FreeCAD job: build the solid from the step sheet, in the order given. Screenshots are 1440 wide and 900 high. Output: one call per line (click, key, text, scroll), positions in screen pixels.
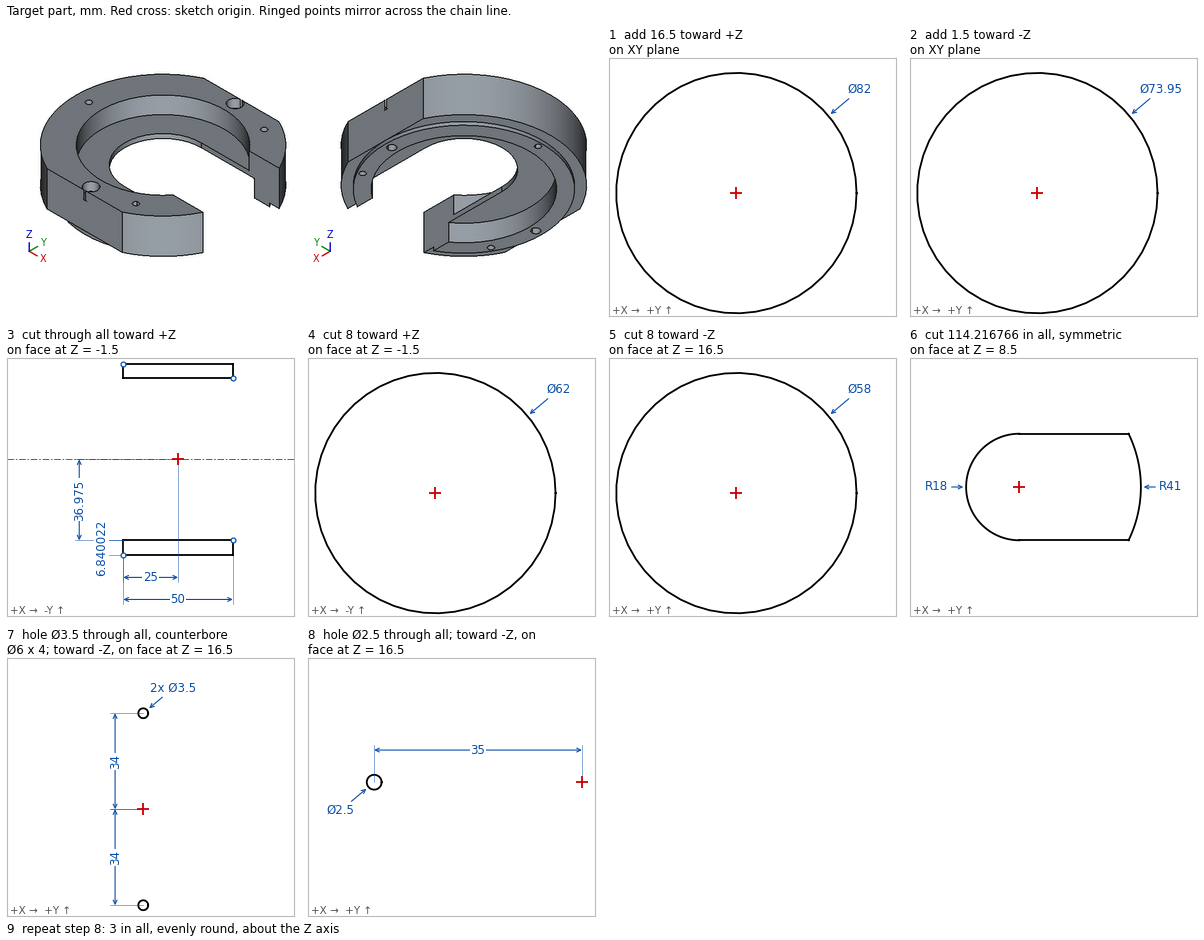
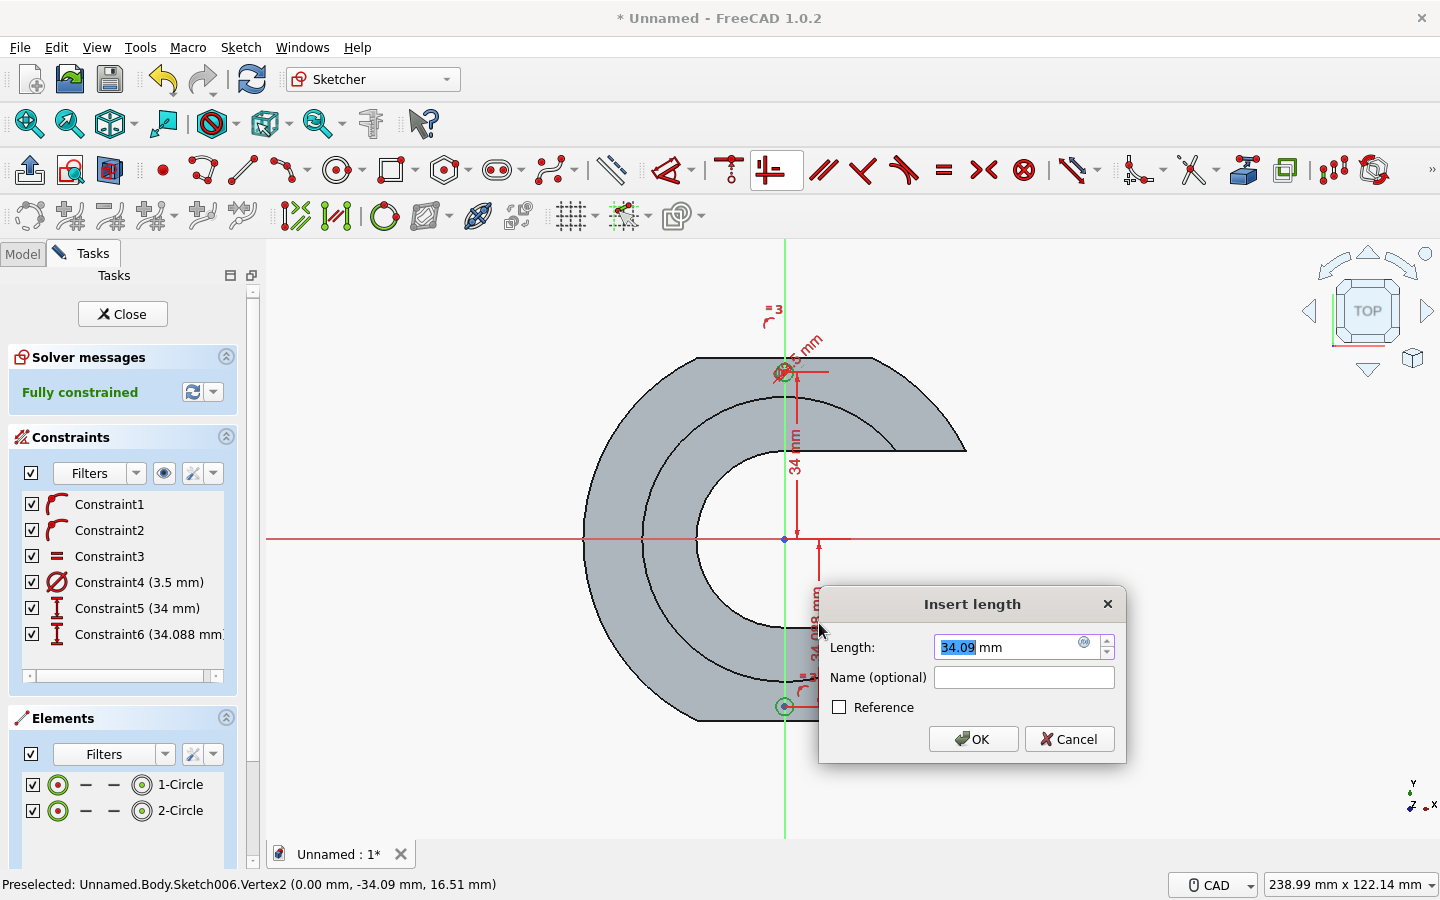
text(34)
key(Return)
key(Escape)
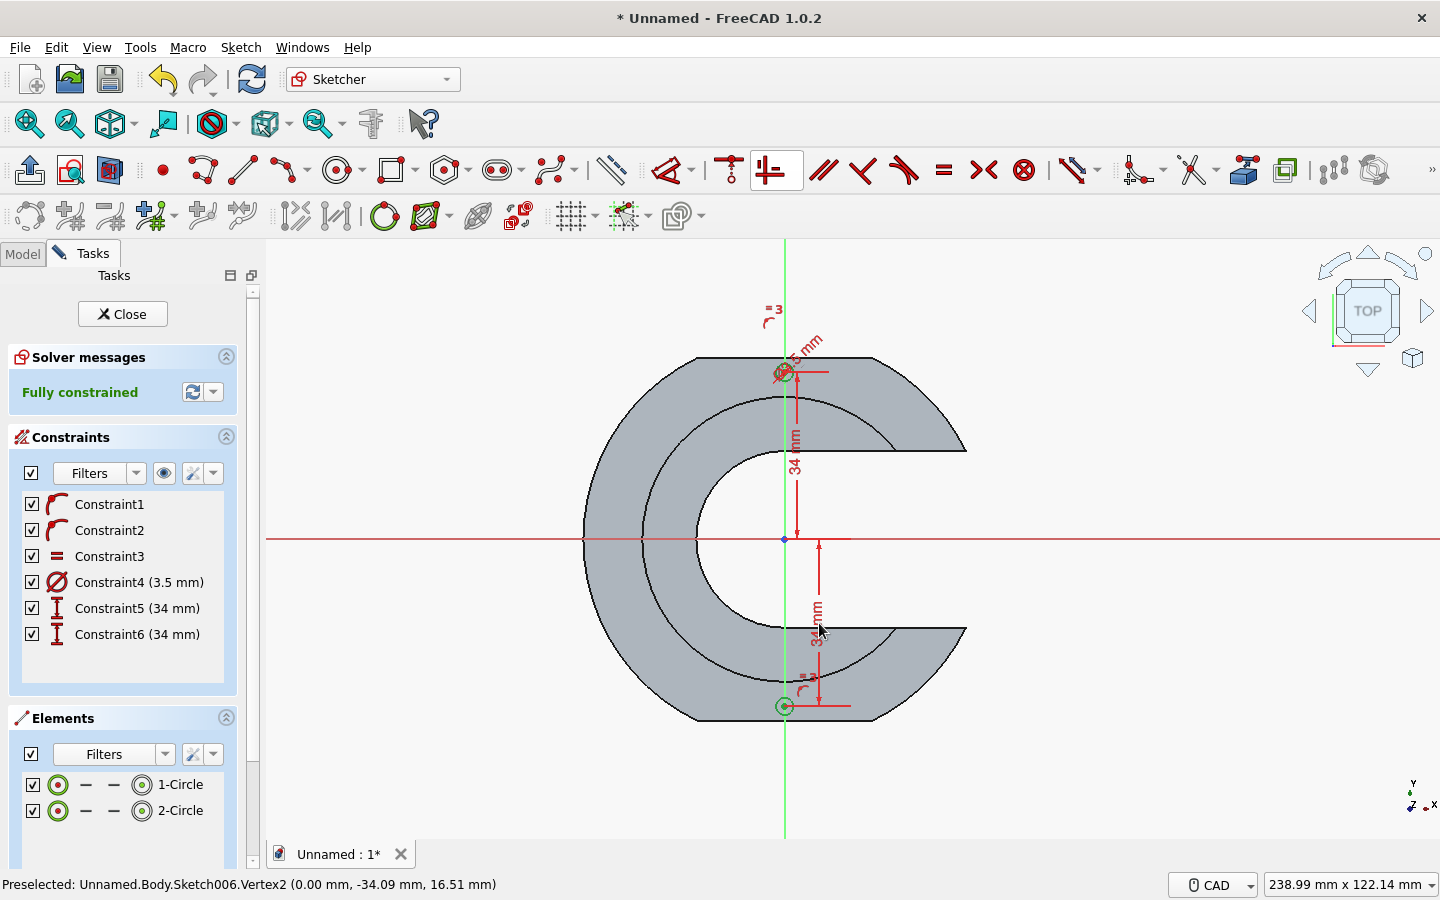
click(123, 314)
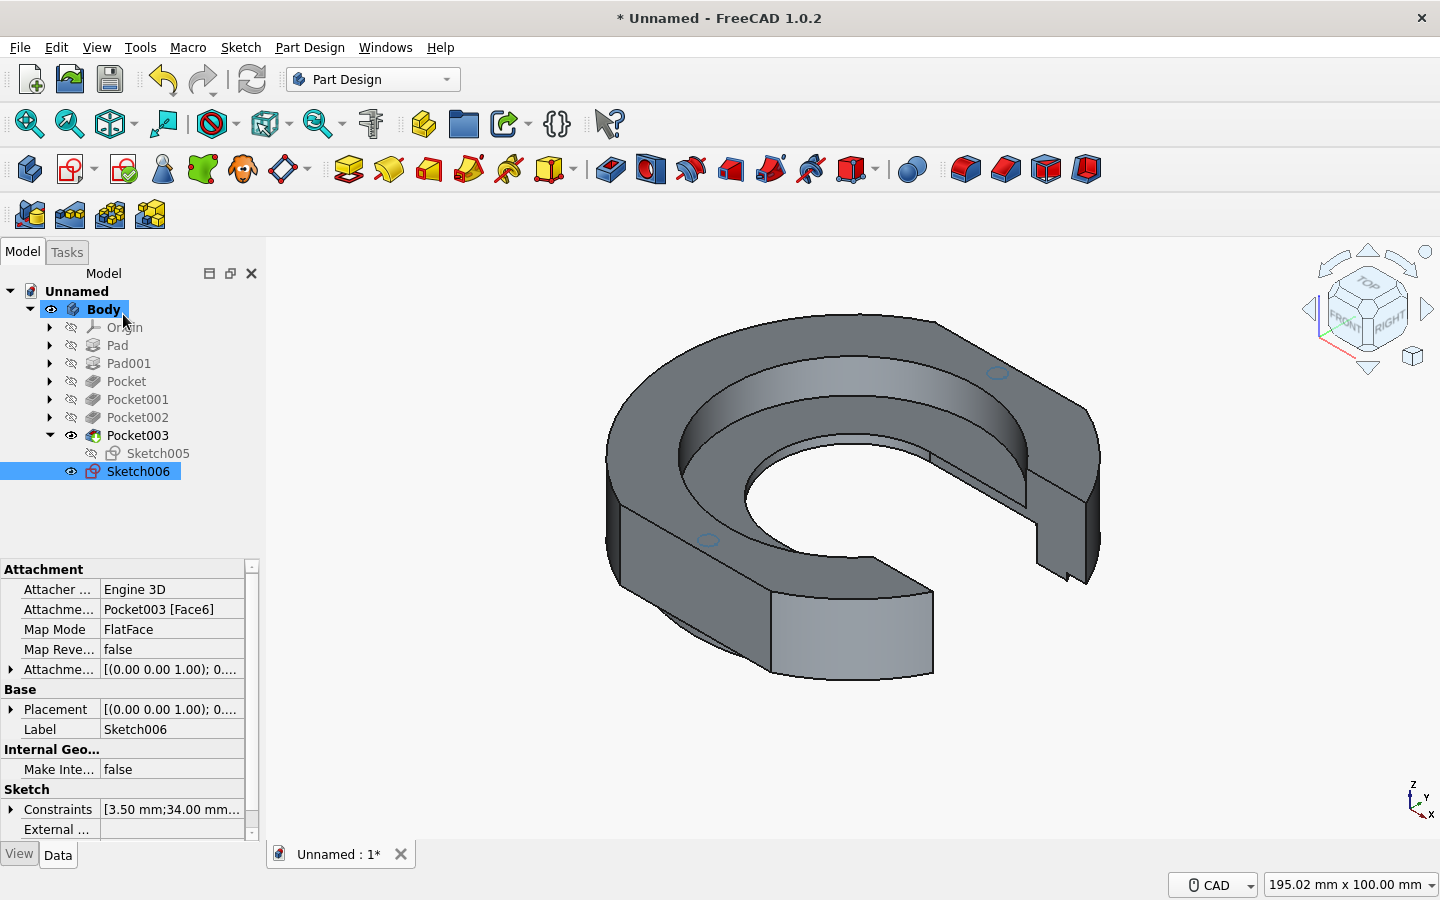
click(652, 170)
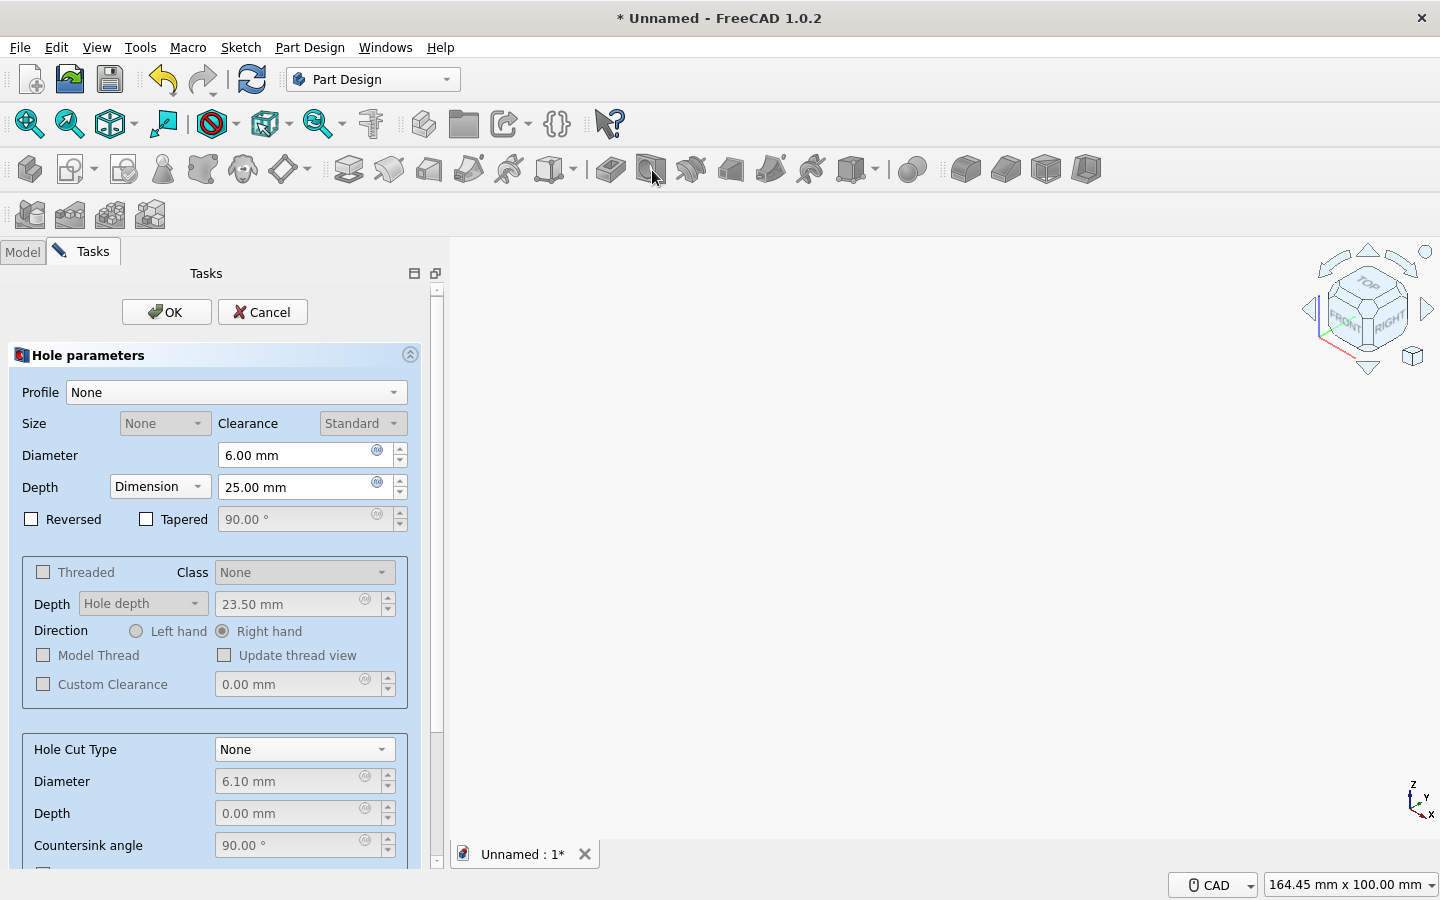
triple_click(305, 455)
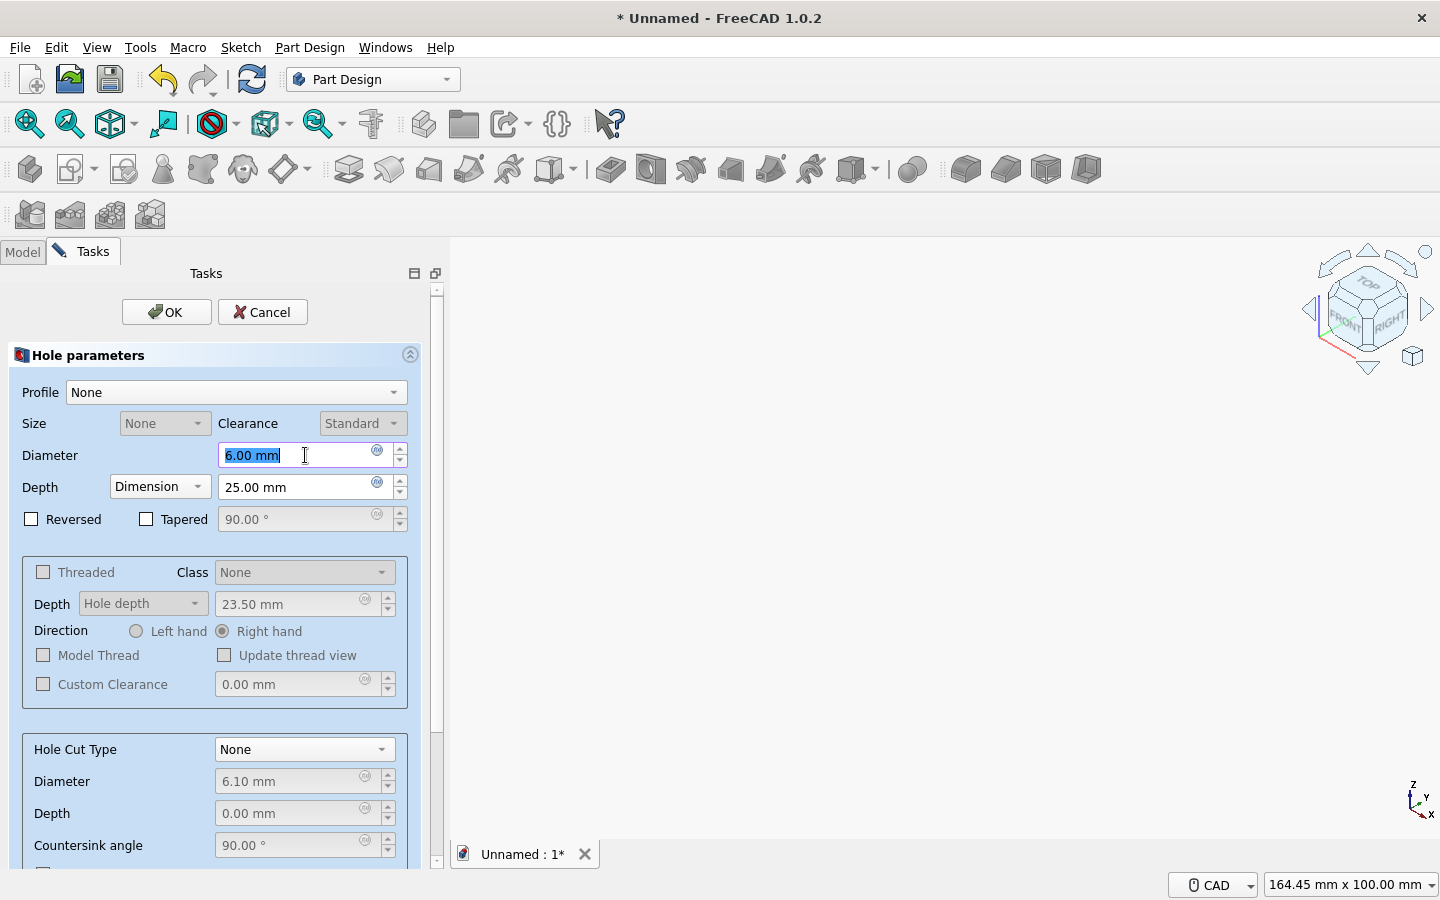
text(3.5)
key(Tab)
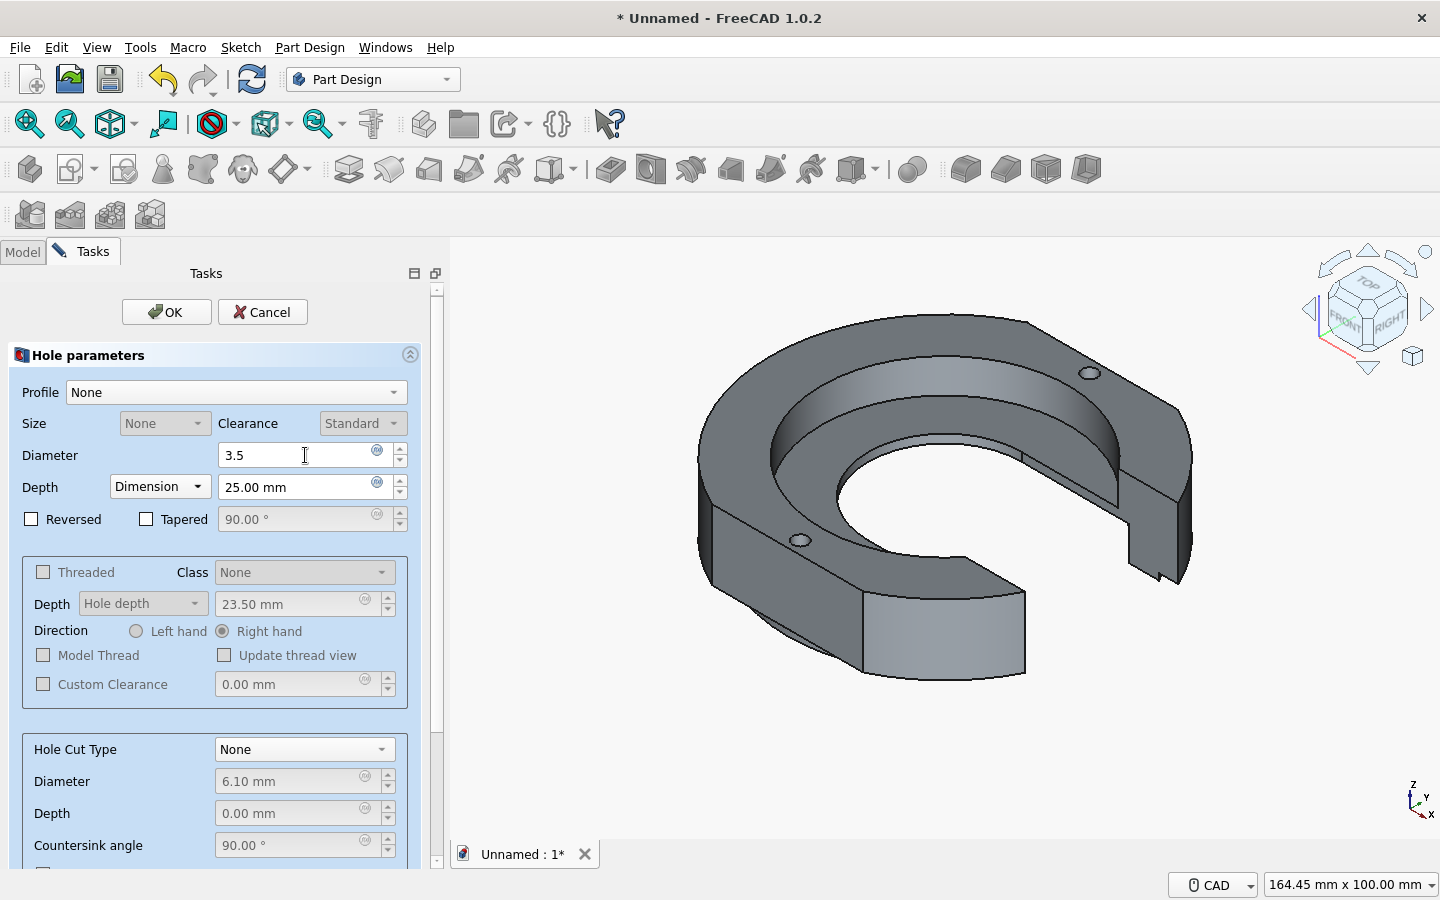
click(161, 486)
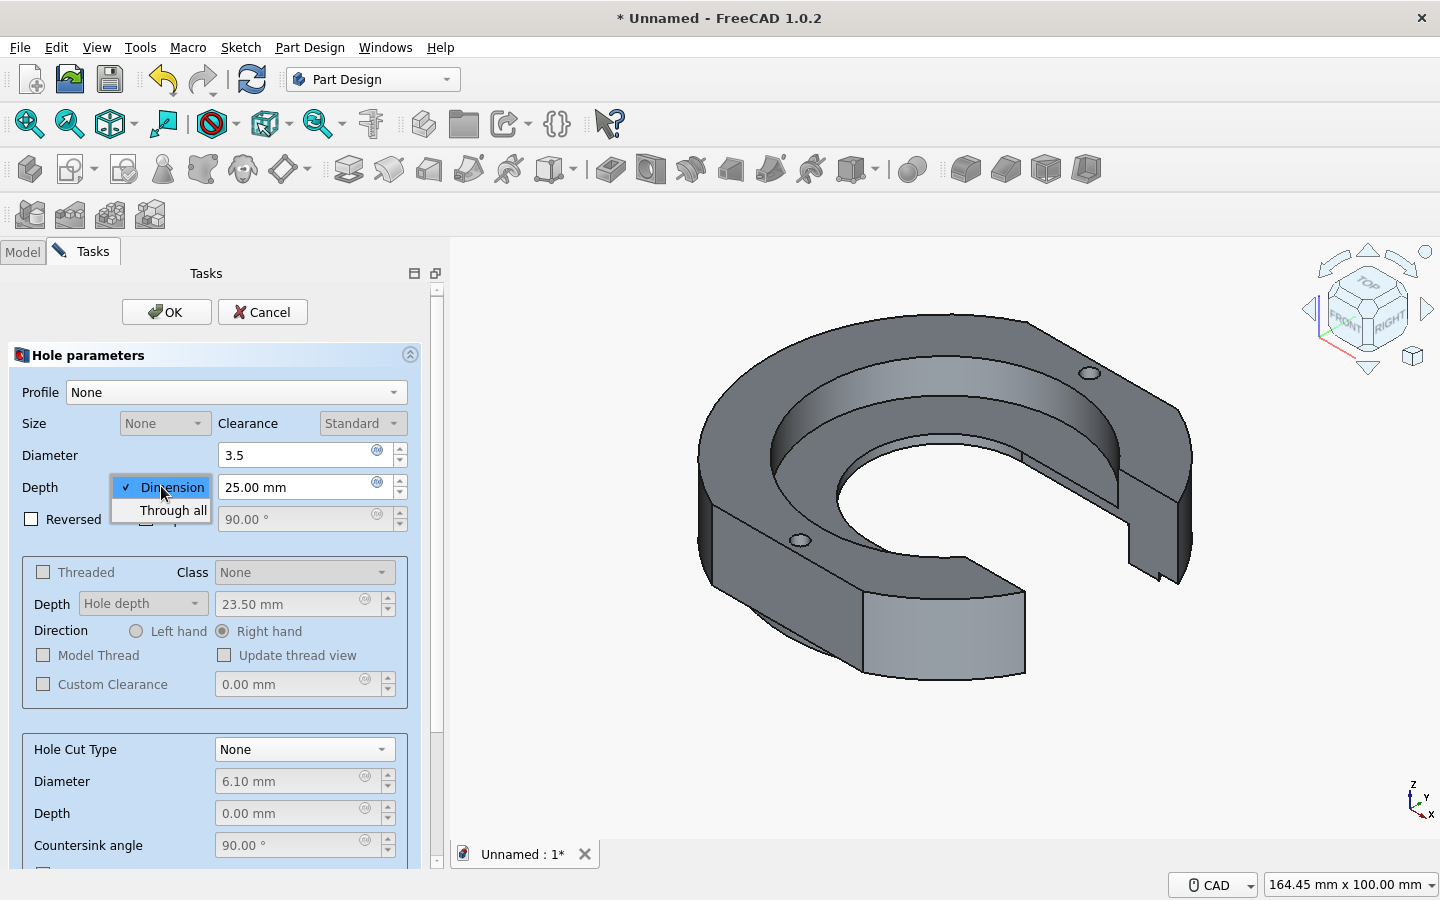
click(160, 510)